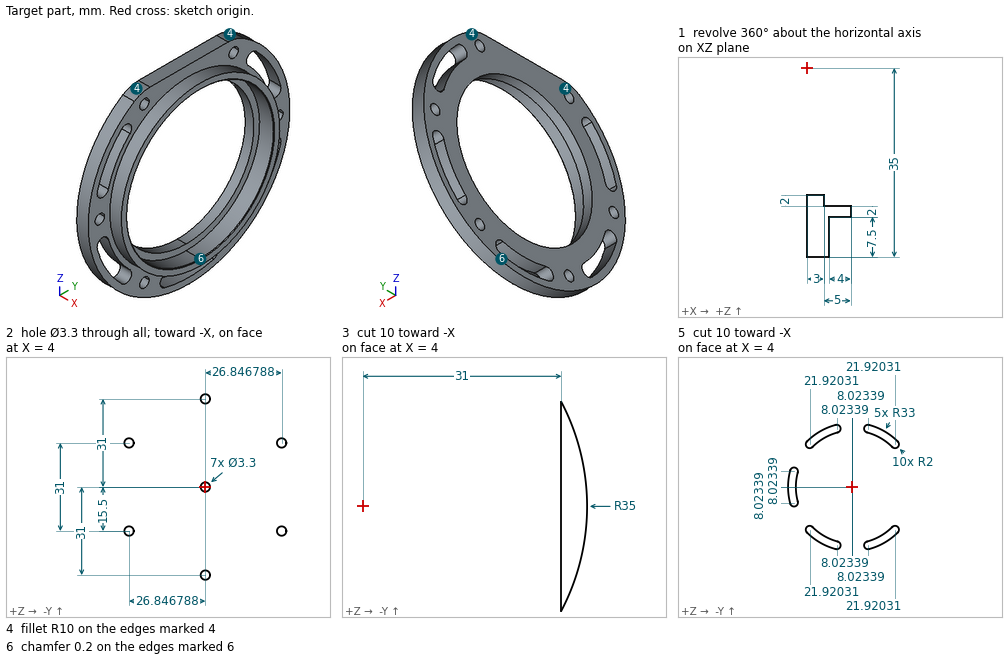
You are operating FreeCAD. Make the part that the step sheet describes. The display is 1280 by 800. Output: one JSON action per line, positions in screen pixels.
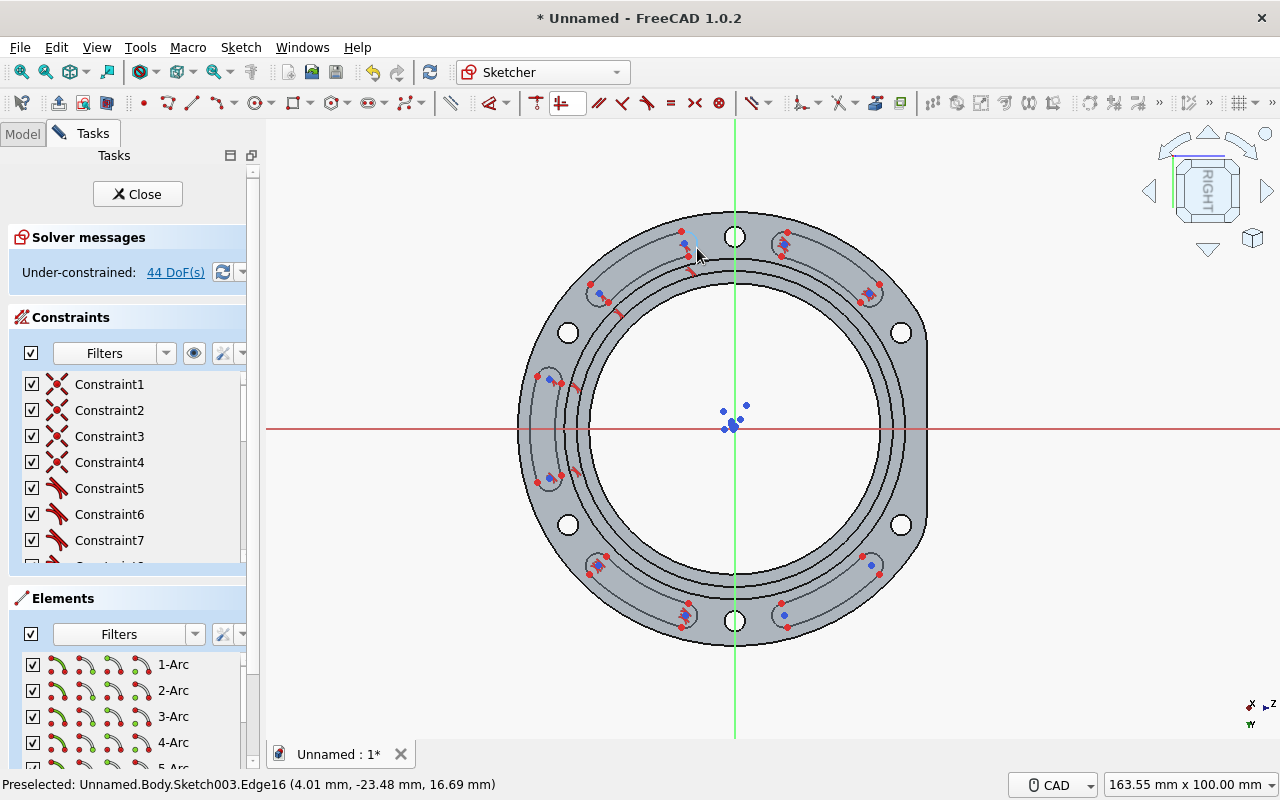
{"action": "left_click", "coordinate": [808, 594]}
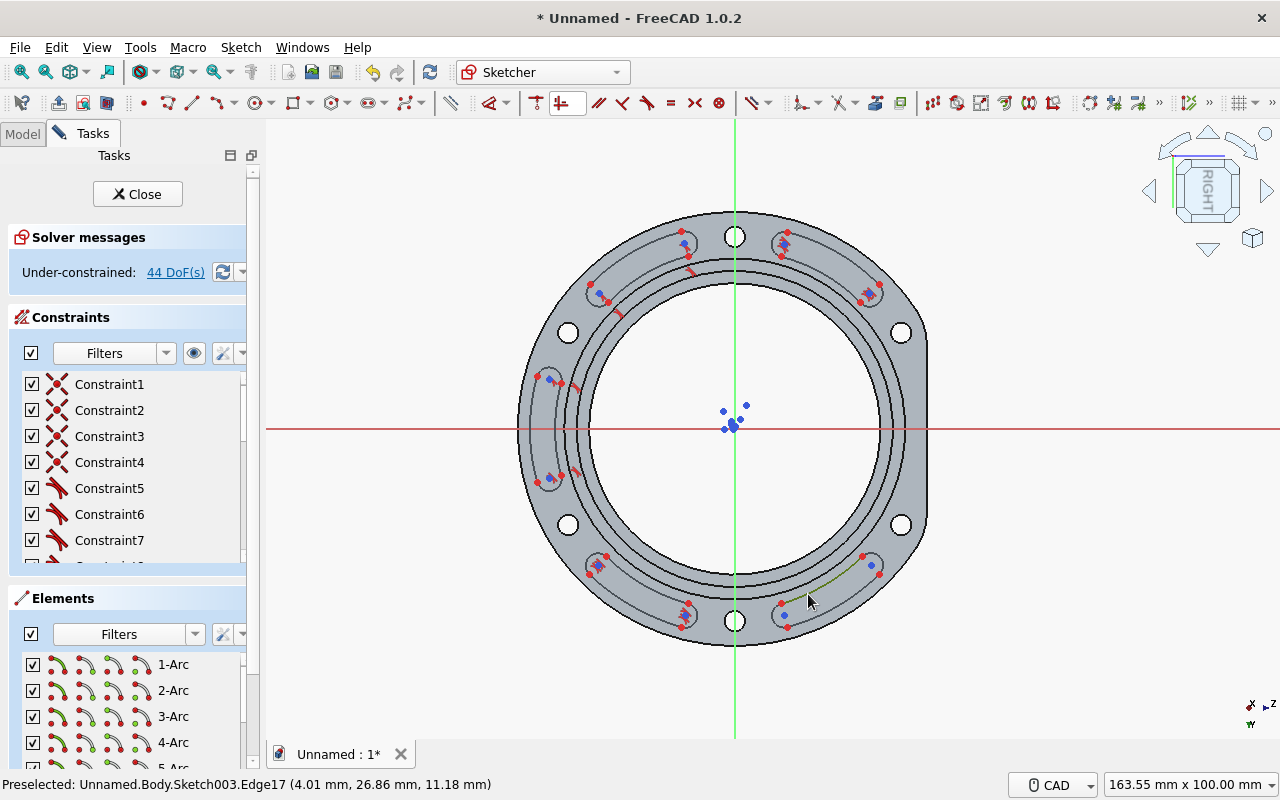
{"action": "scroll", "coordinate": [773, 611], "scroll_direction": "up", "scroll_amount": 2}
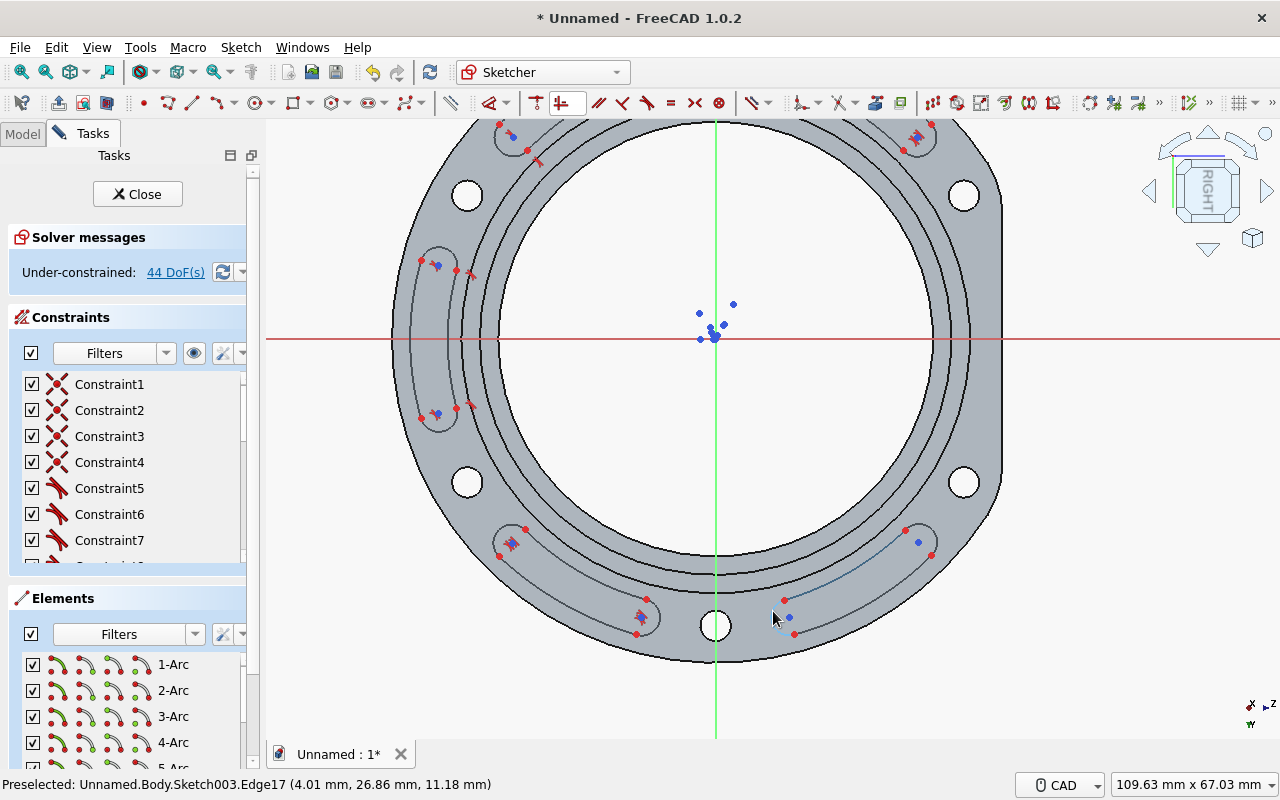
{"action": "left_click", "coordinate": [772, 611]}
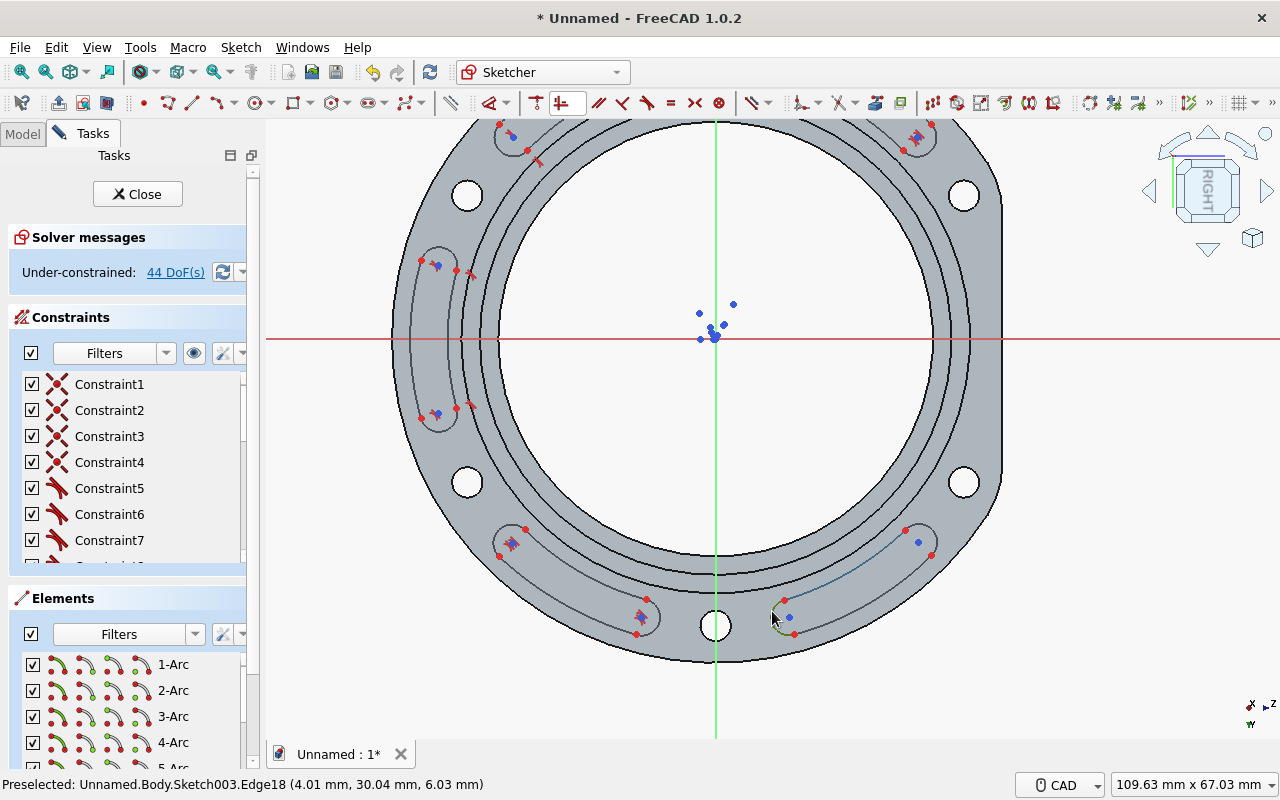
{"action": "left_click", "coordinate": [648, 104]}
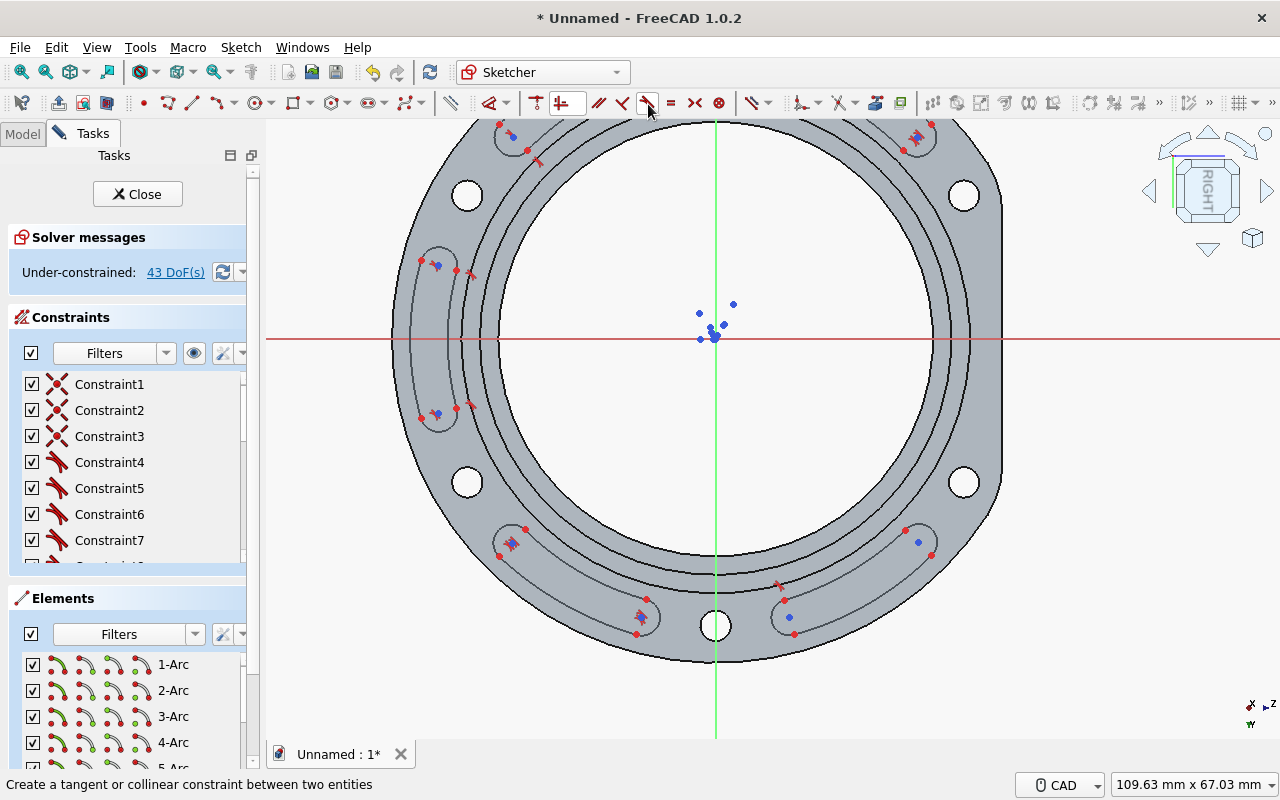
{"action": "left_click", "coordinate": [824, 585]}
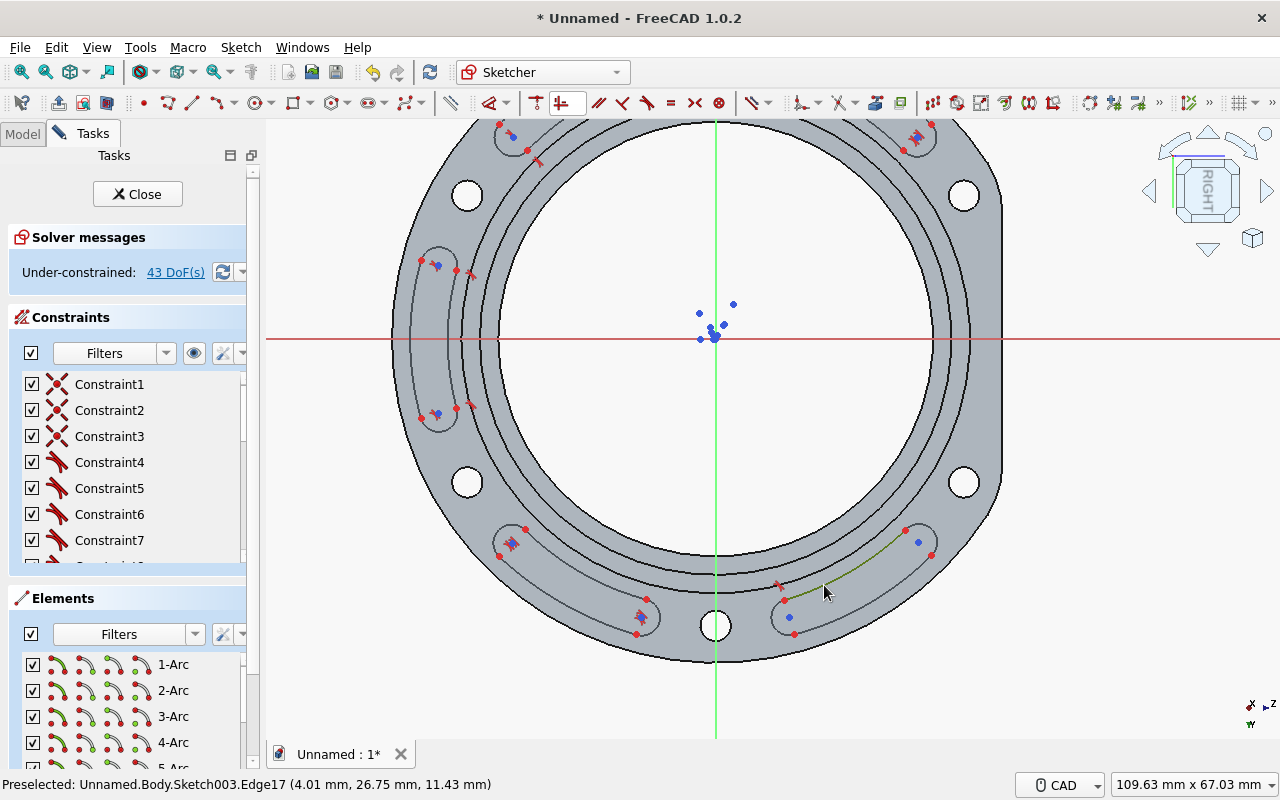
{"action": "left_click", "coordinate": [937, 540]}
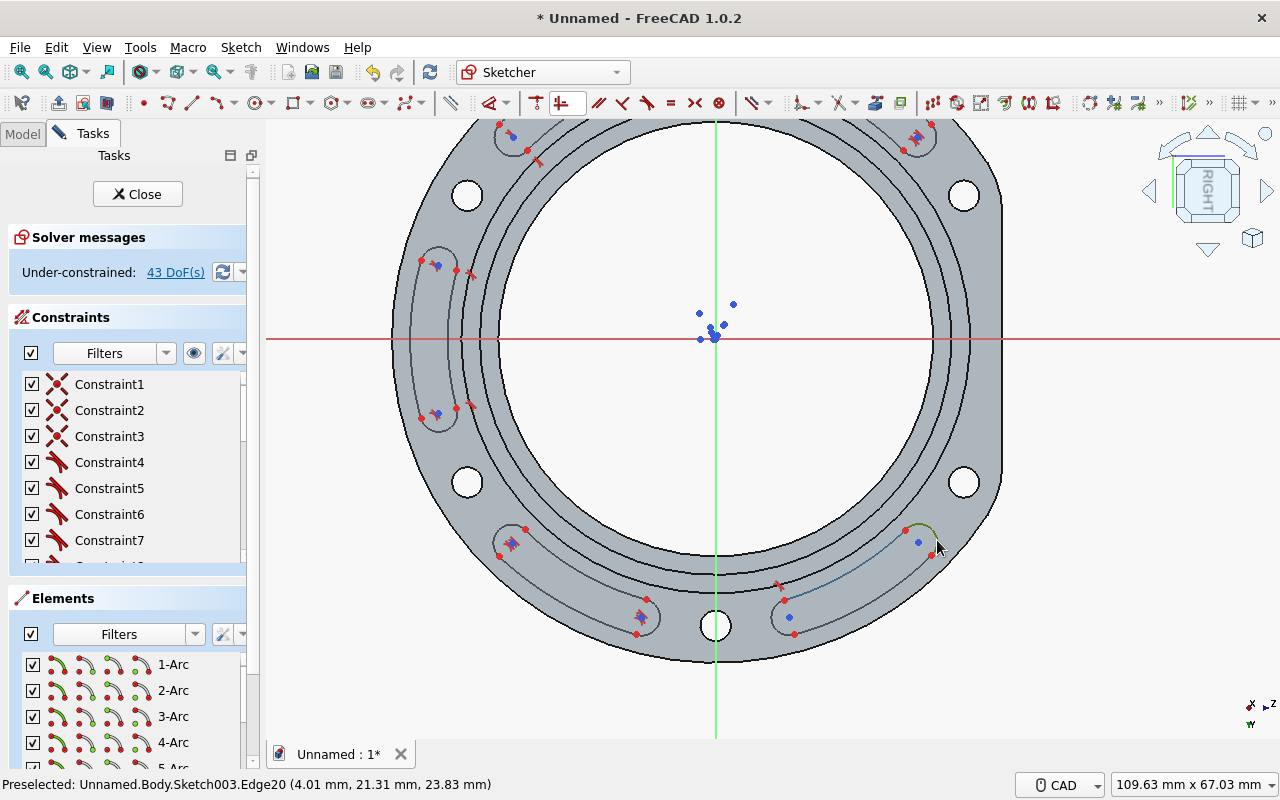
{"action": "left_click", "coordinate": [648, 104]}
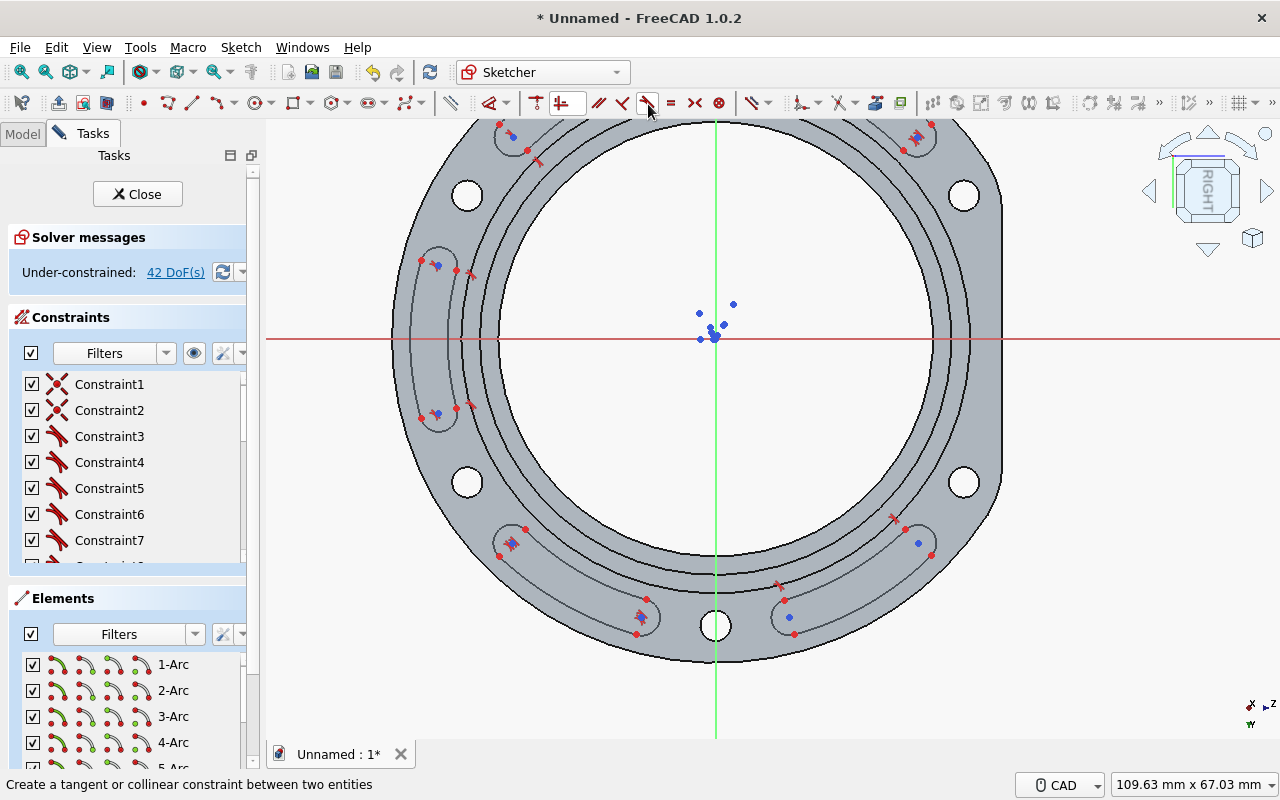
{"action": "left_click", "coordinate": [772, 612]}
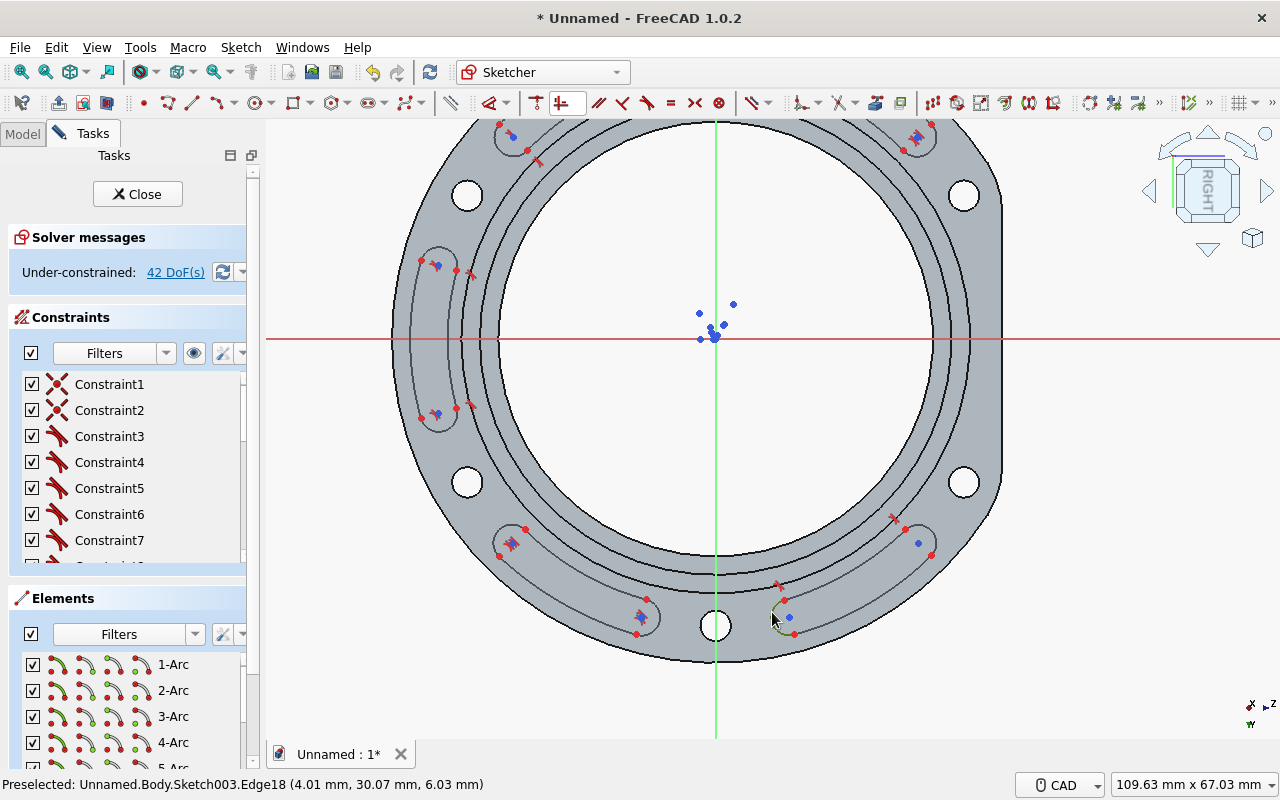
{"action": "left_click", "coordinate": [840, 618]}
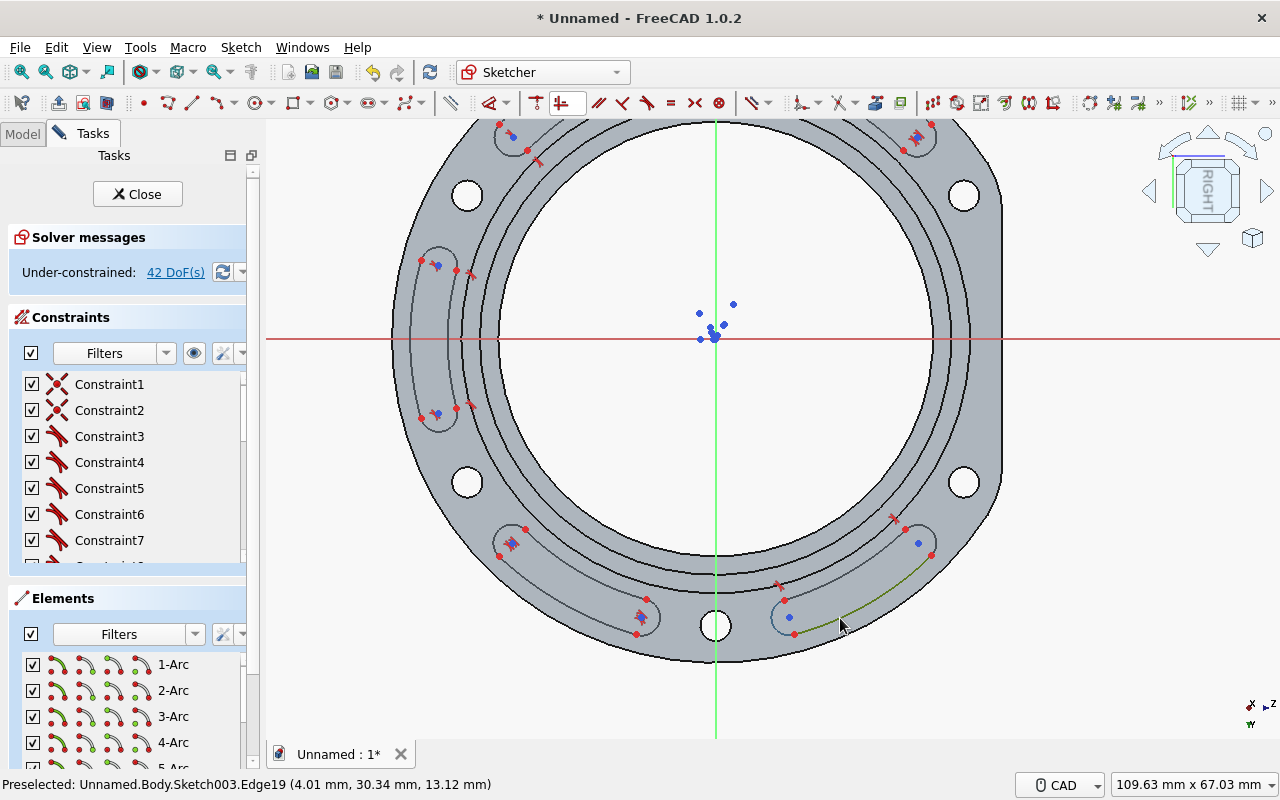
{"action": "left_click", "coordinate": [648, 104]}